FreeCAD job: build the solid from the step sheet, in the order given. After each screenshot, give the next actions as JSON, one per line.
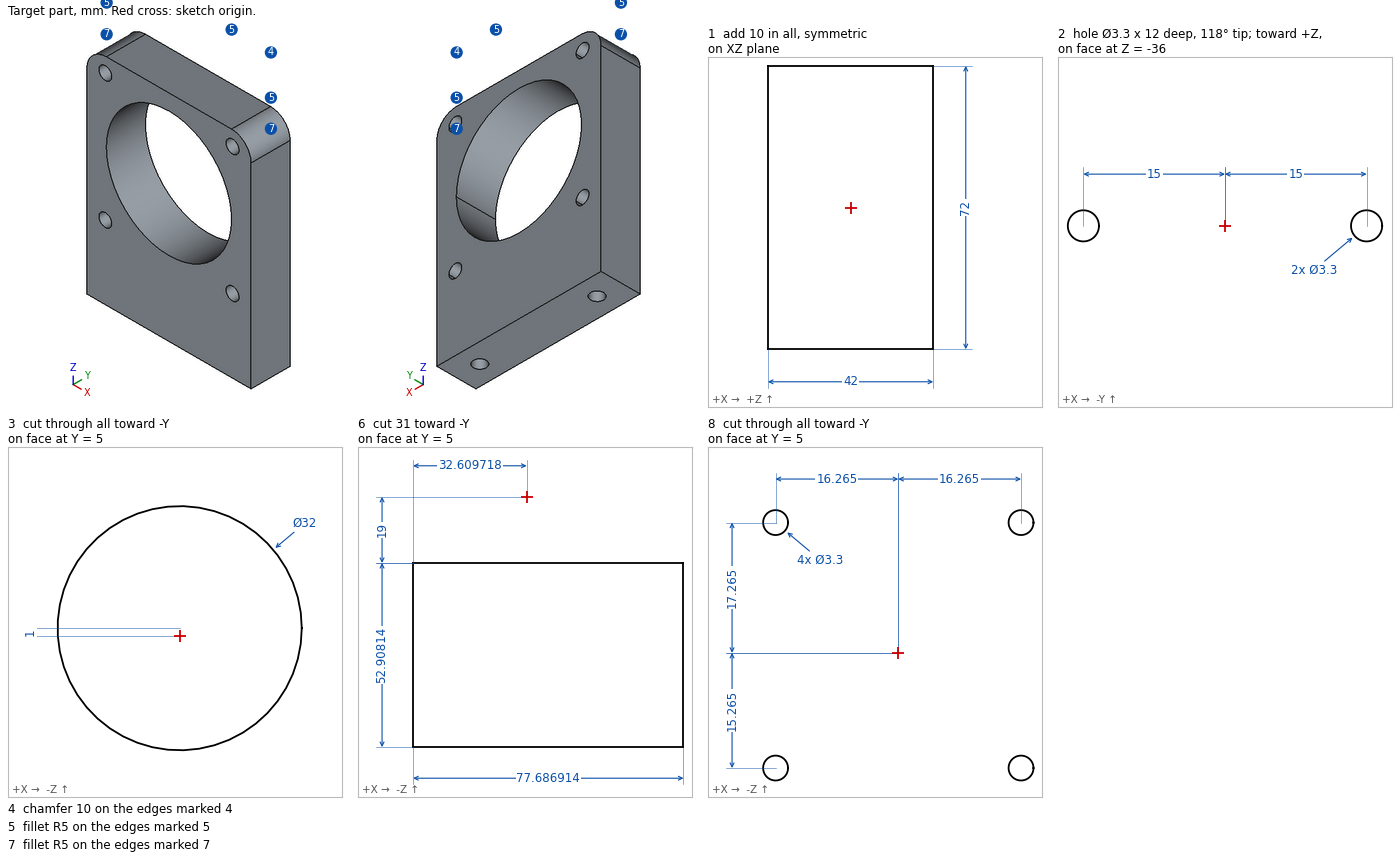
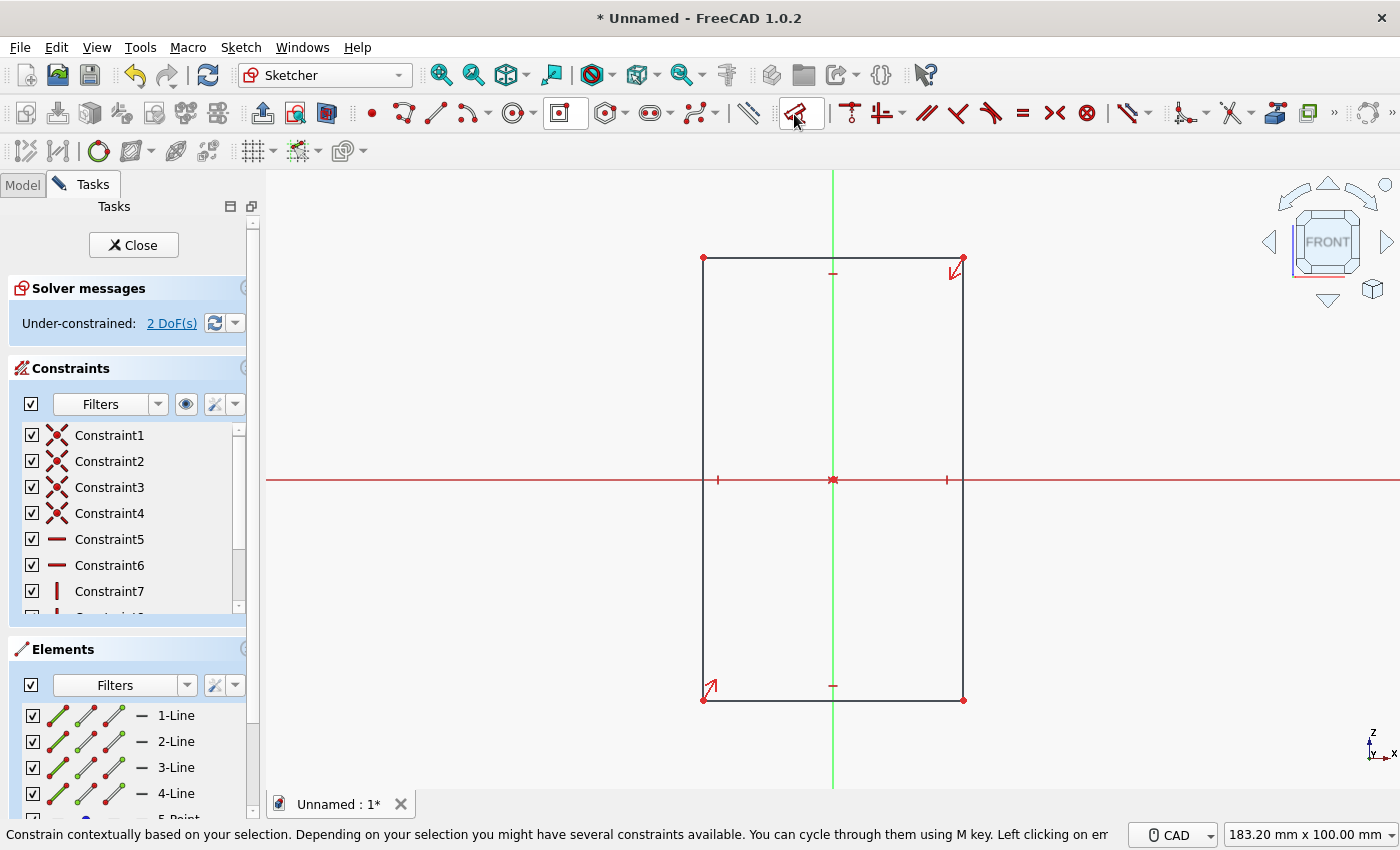
{"action": "left_click", "coordinate": [781, 701]}
{"action": "left_click", "coordinate": [773, 735]}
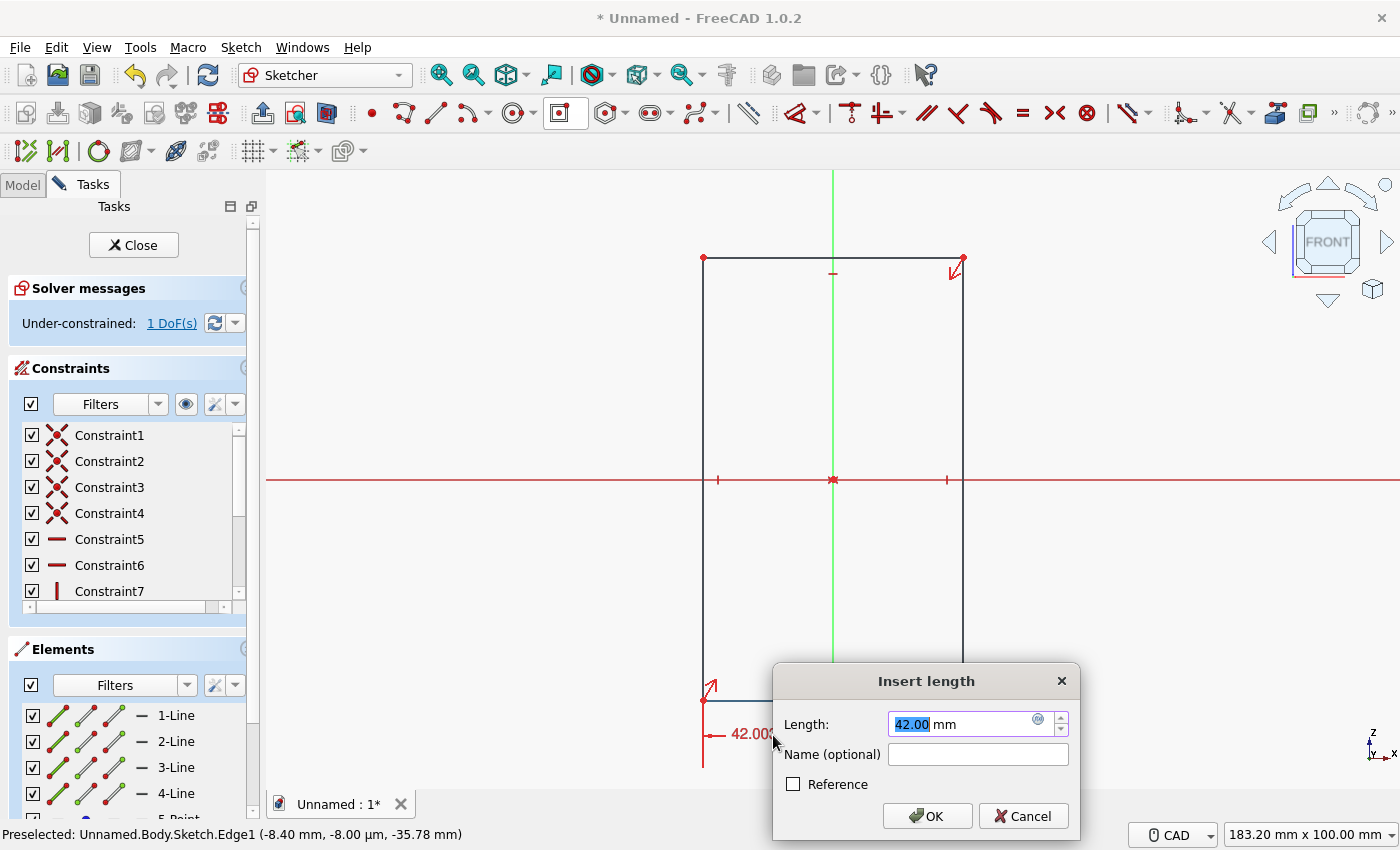
{"action": "type", "text": "42"}
{"action": "key", "text": "Return"}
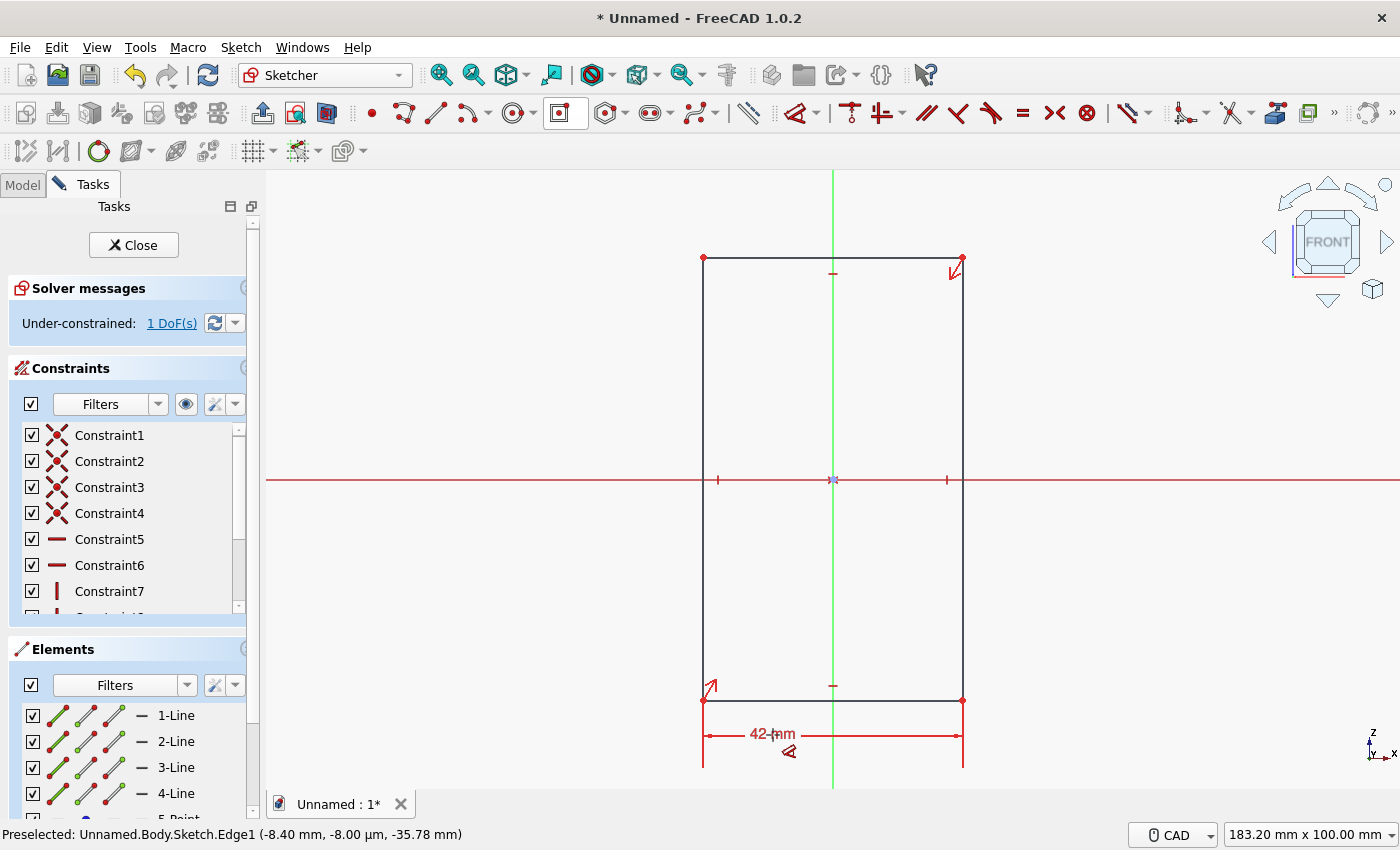
{"action": "left_click", "coordinate": [963, 568]}
{"action": "left_click", "coordinate": [997, 378]}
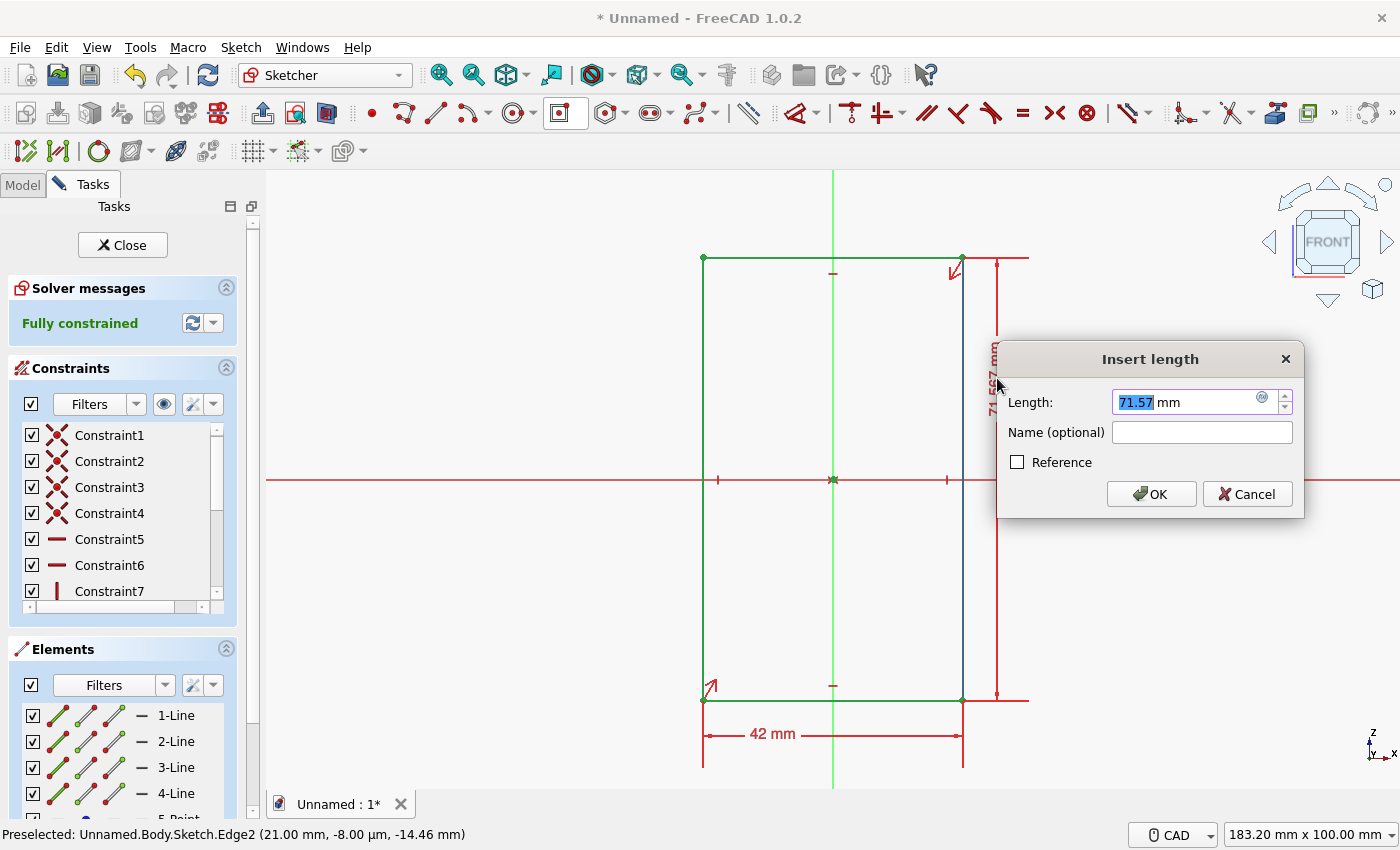
{"action": "type", "text": "72"}
{"action": "key", "text": "Return"}
{"action": "key", "text": "Escape"}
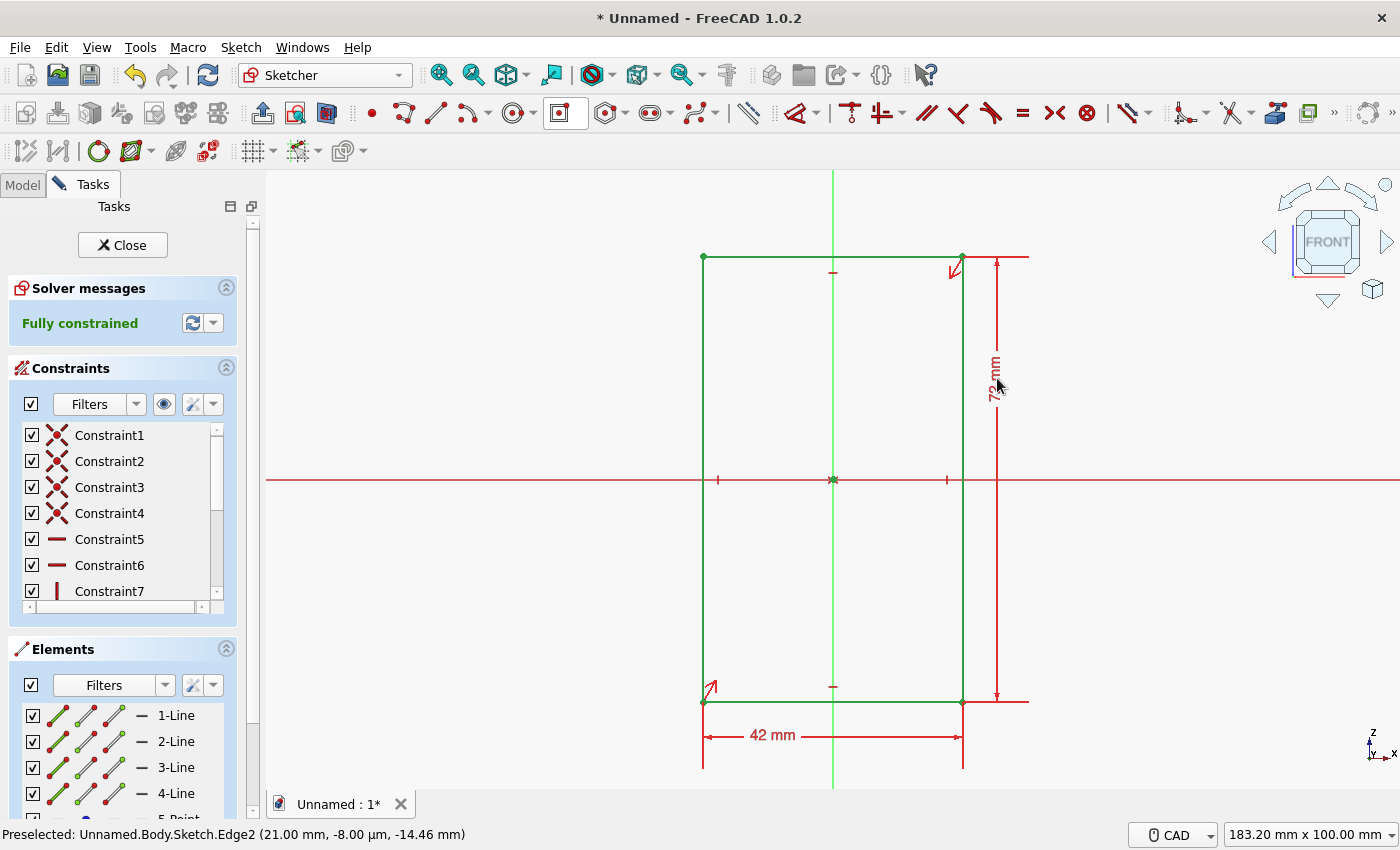
{"action": "left_click", "coordinate": [123, 245]}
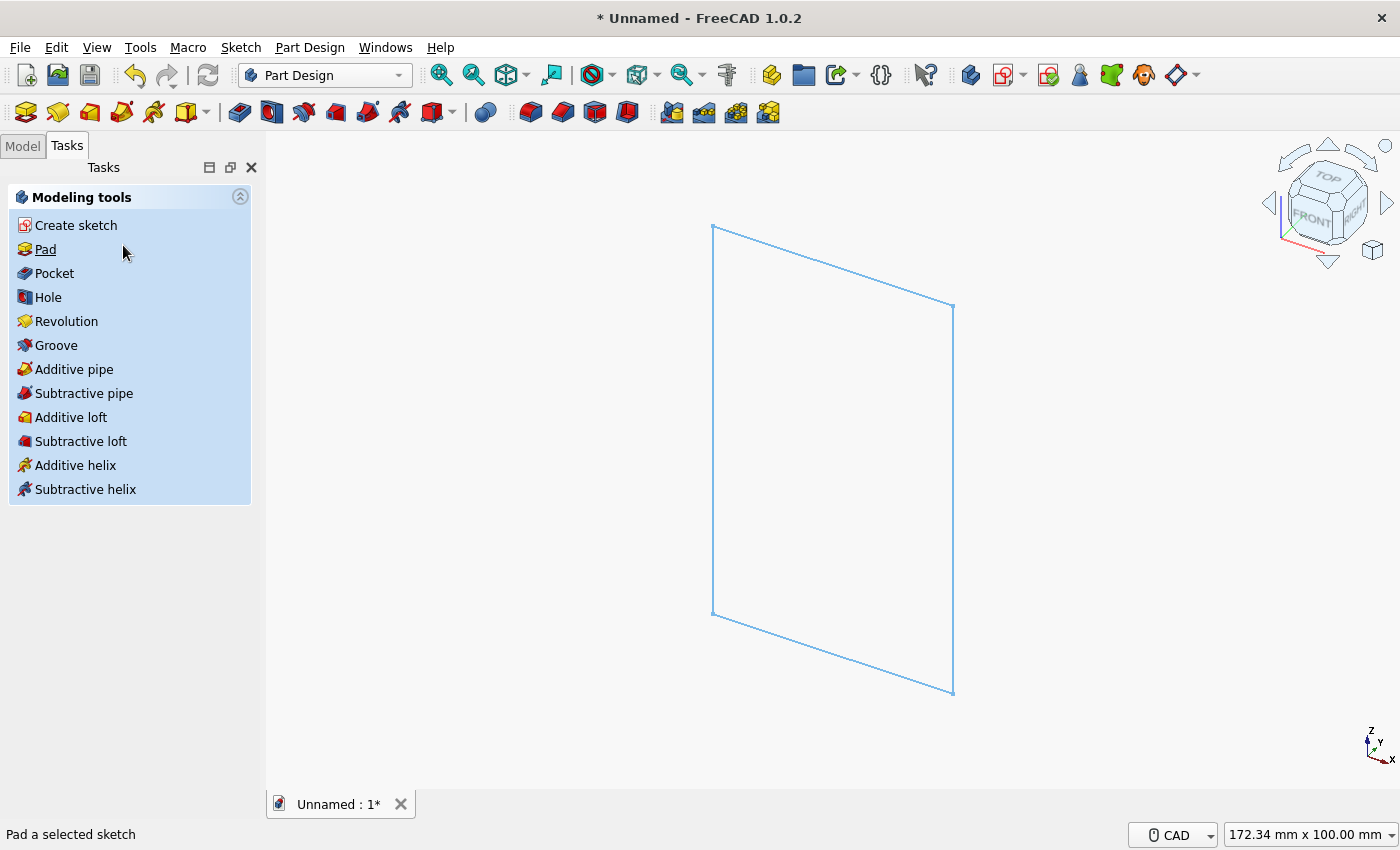
{"action": "left_click", "coordinate": [26, 112]}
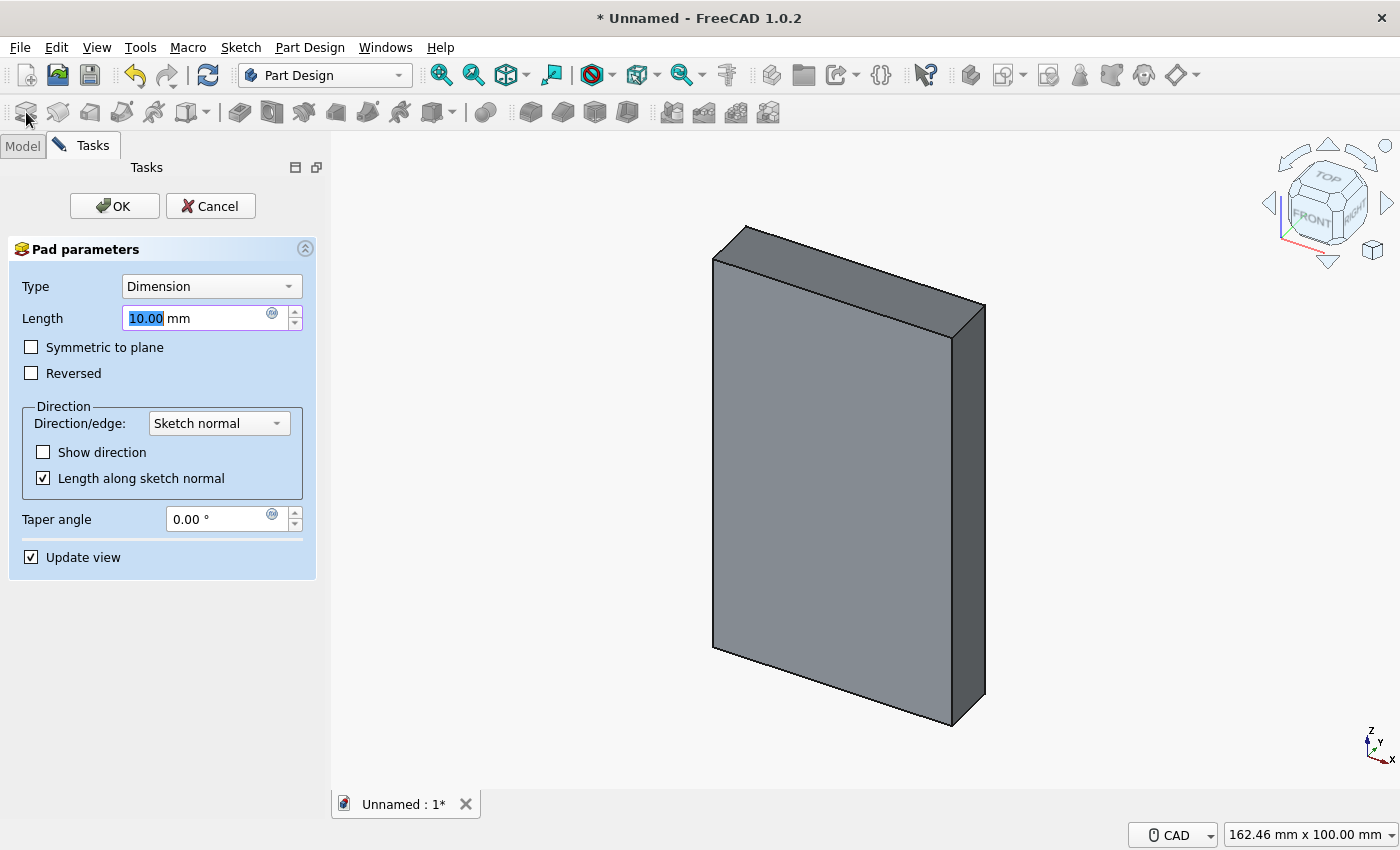
{"action": "type", "text": "10"}
{"action": "key", "text": "Tab"}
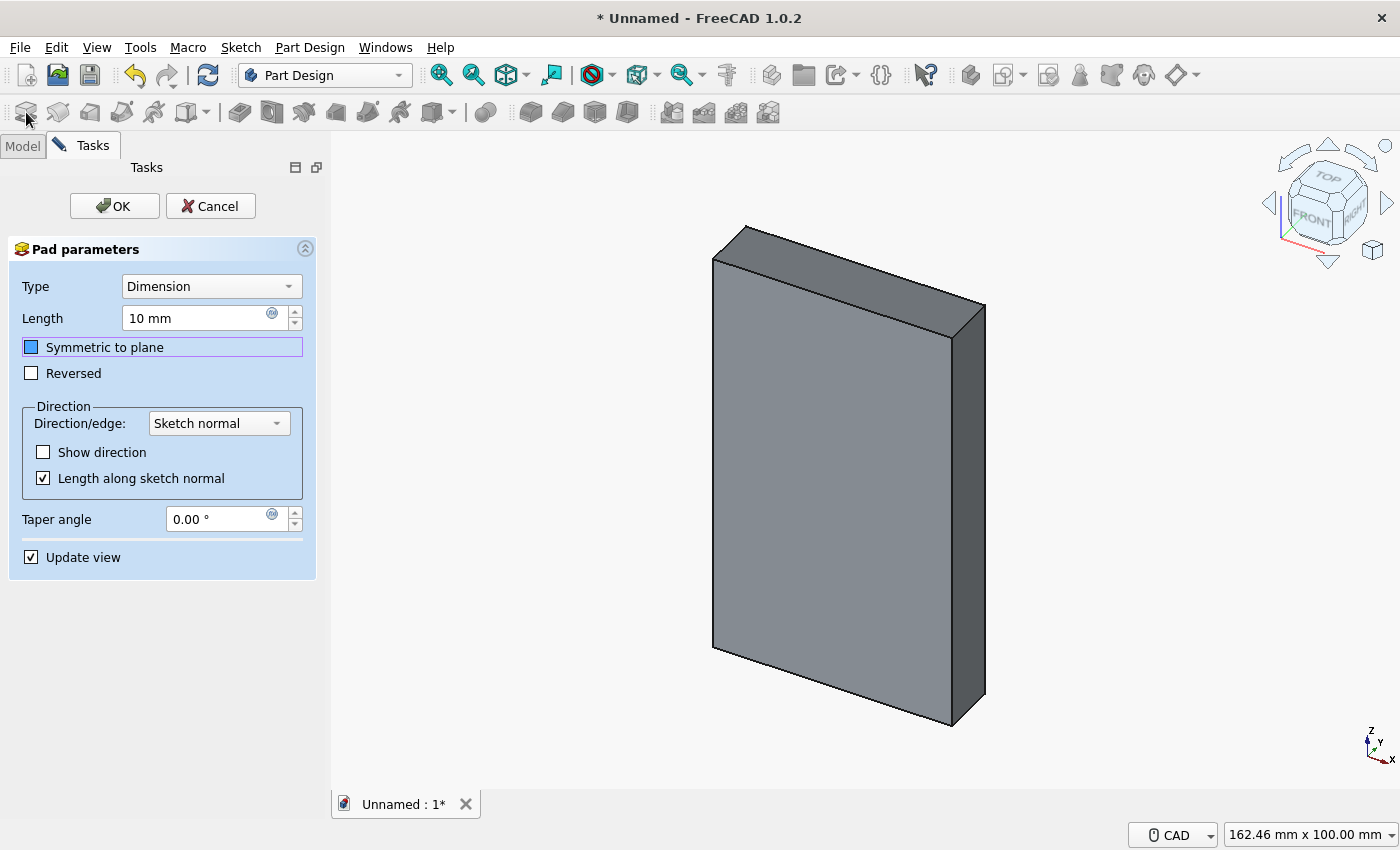
{"action": "left_click", "coordinate": [30, 347]}